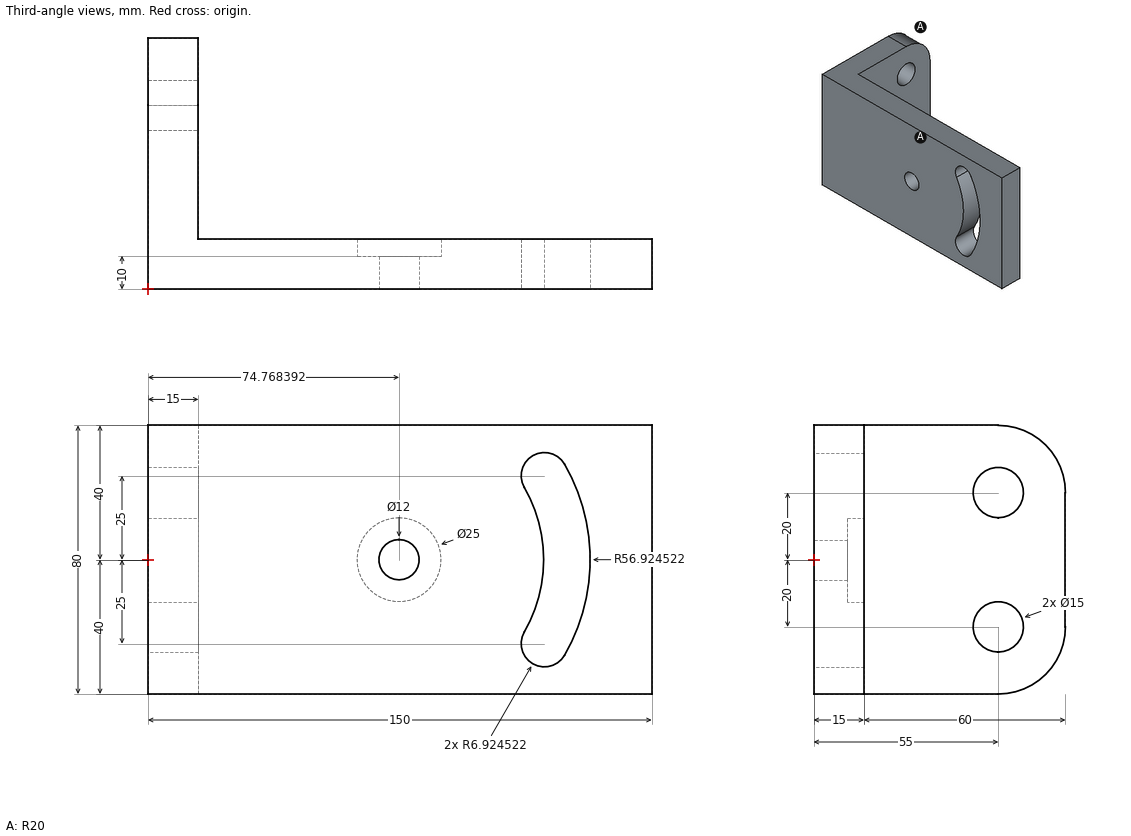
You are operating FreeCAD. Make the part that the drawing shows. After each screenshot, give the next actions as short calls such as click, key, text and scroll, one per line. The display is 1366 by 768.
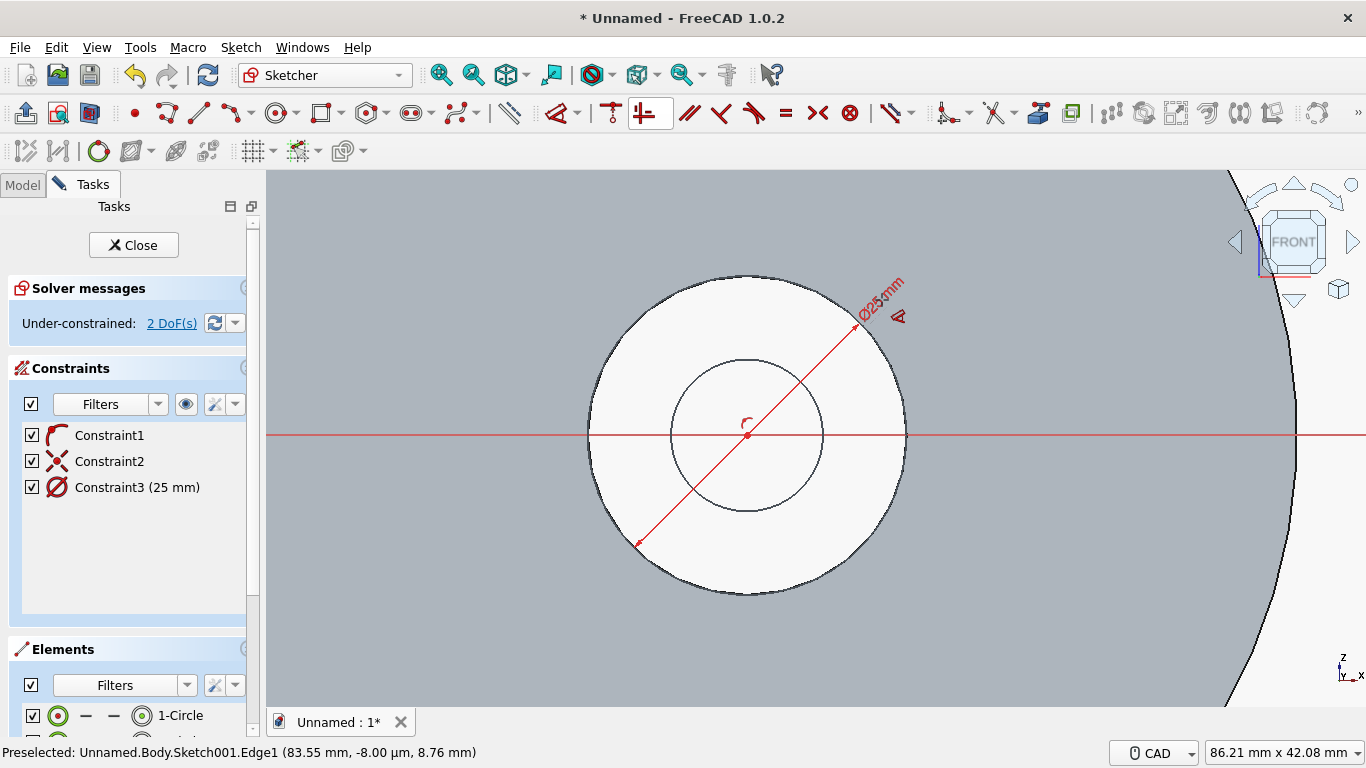
click(801, 382)
click(824, 359)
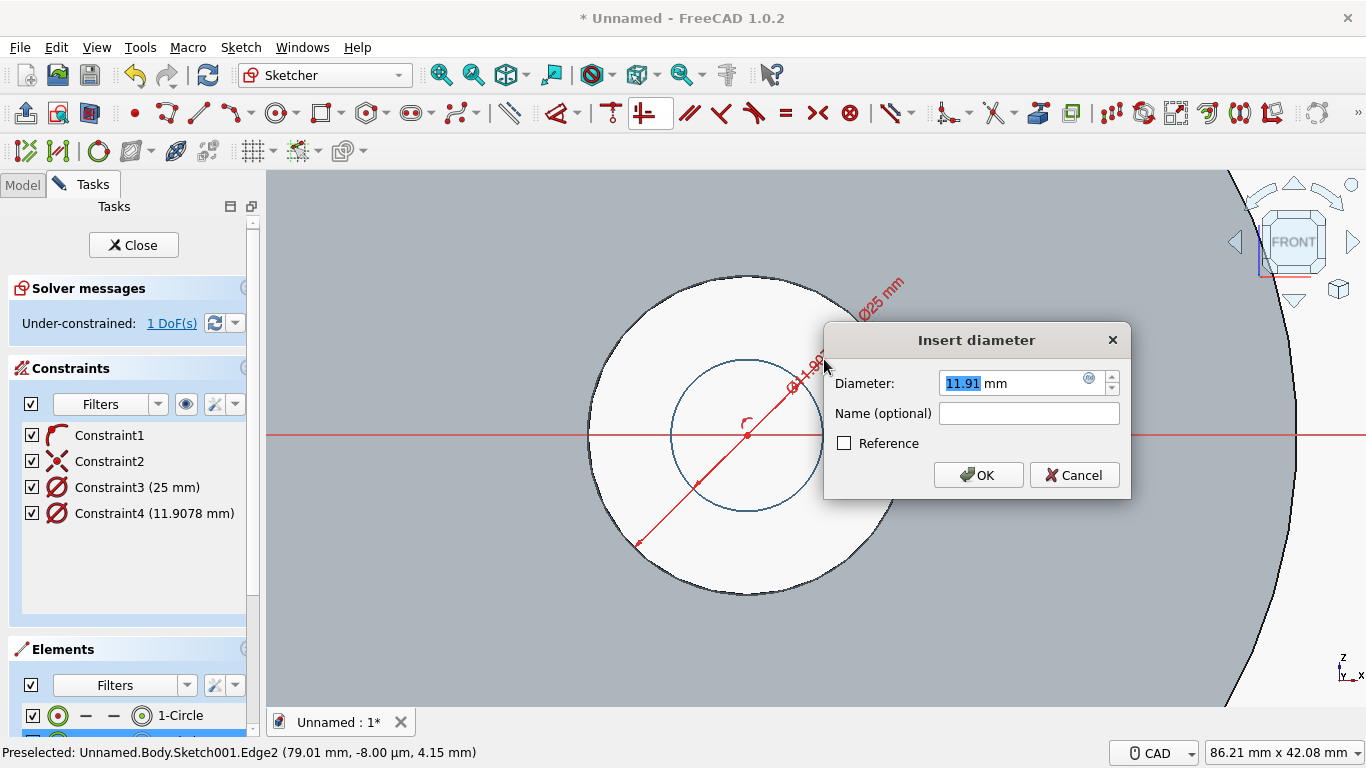
text(12)
key(Return)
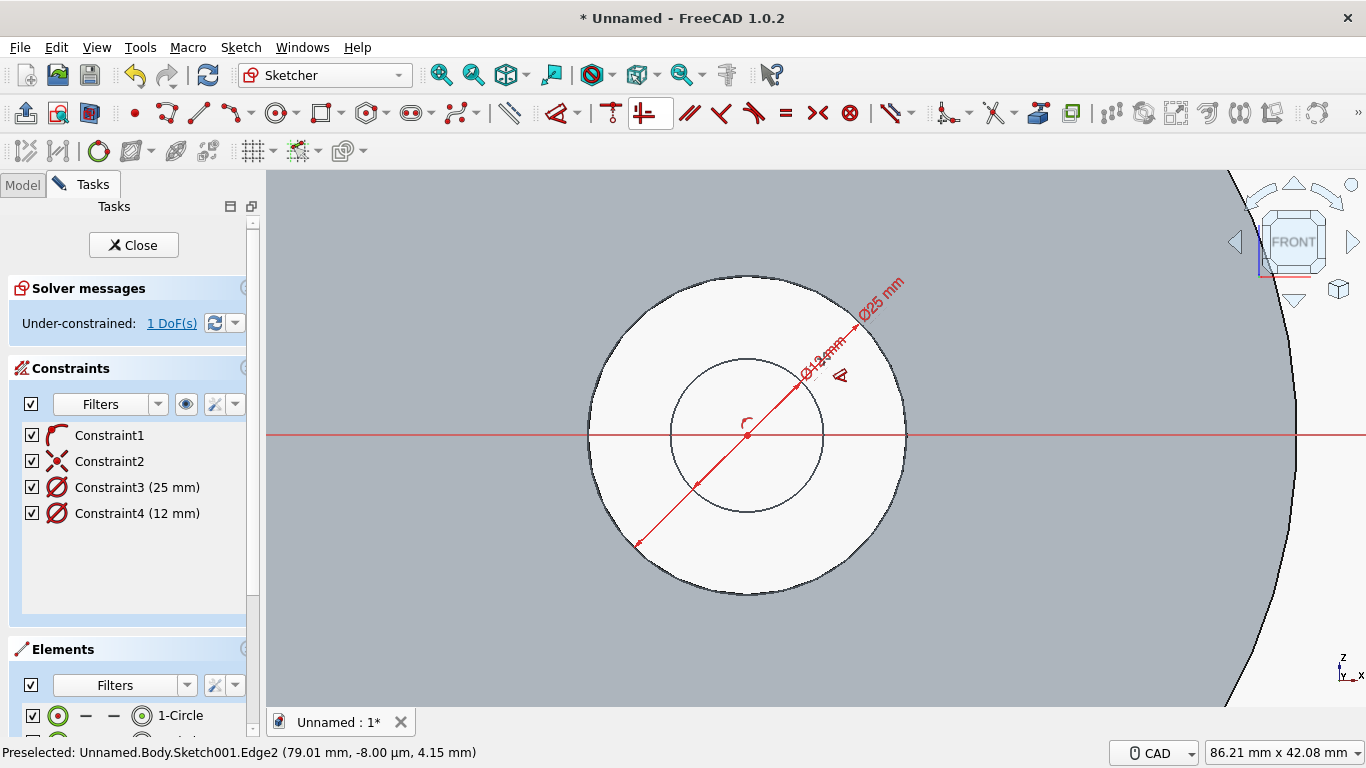
click(747, 435)
click(521, 469)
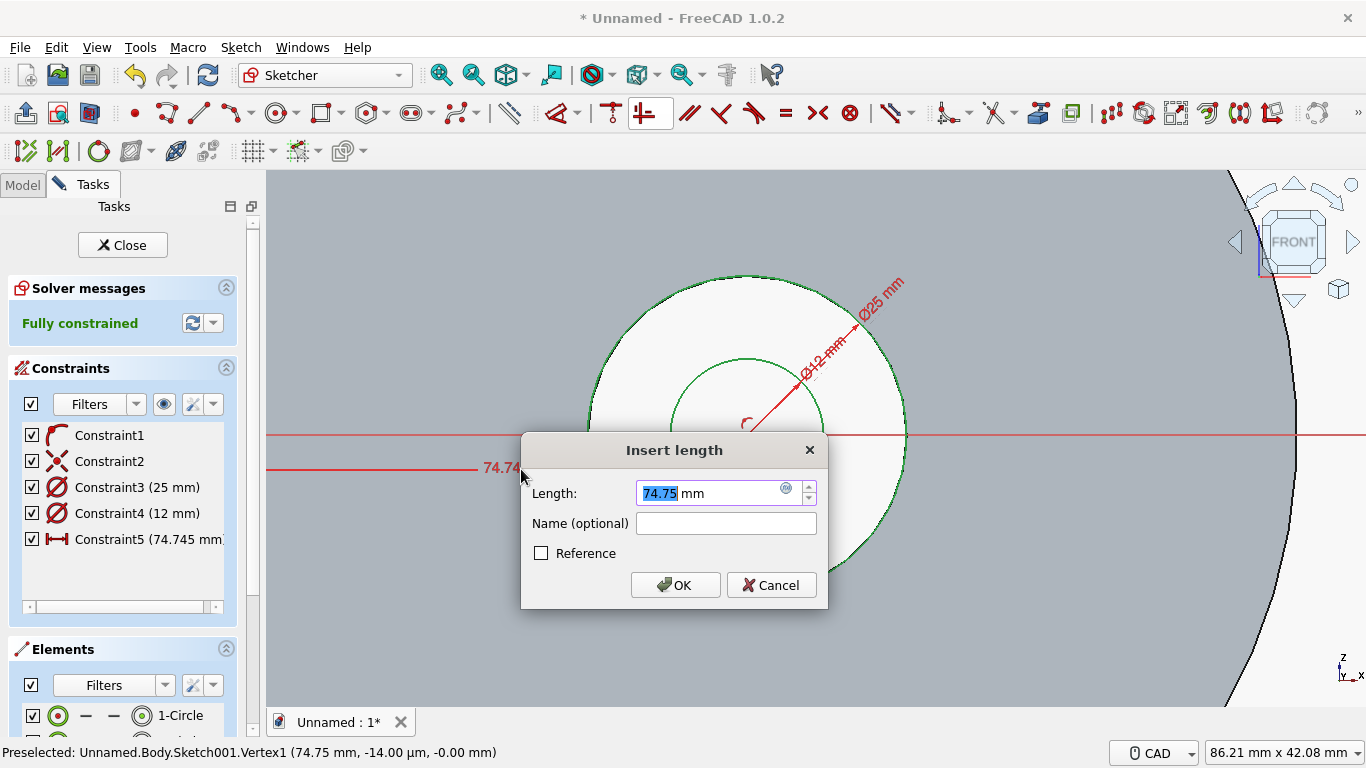
text(74.768392)
key(Return)
key(Escape)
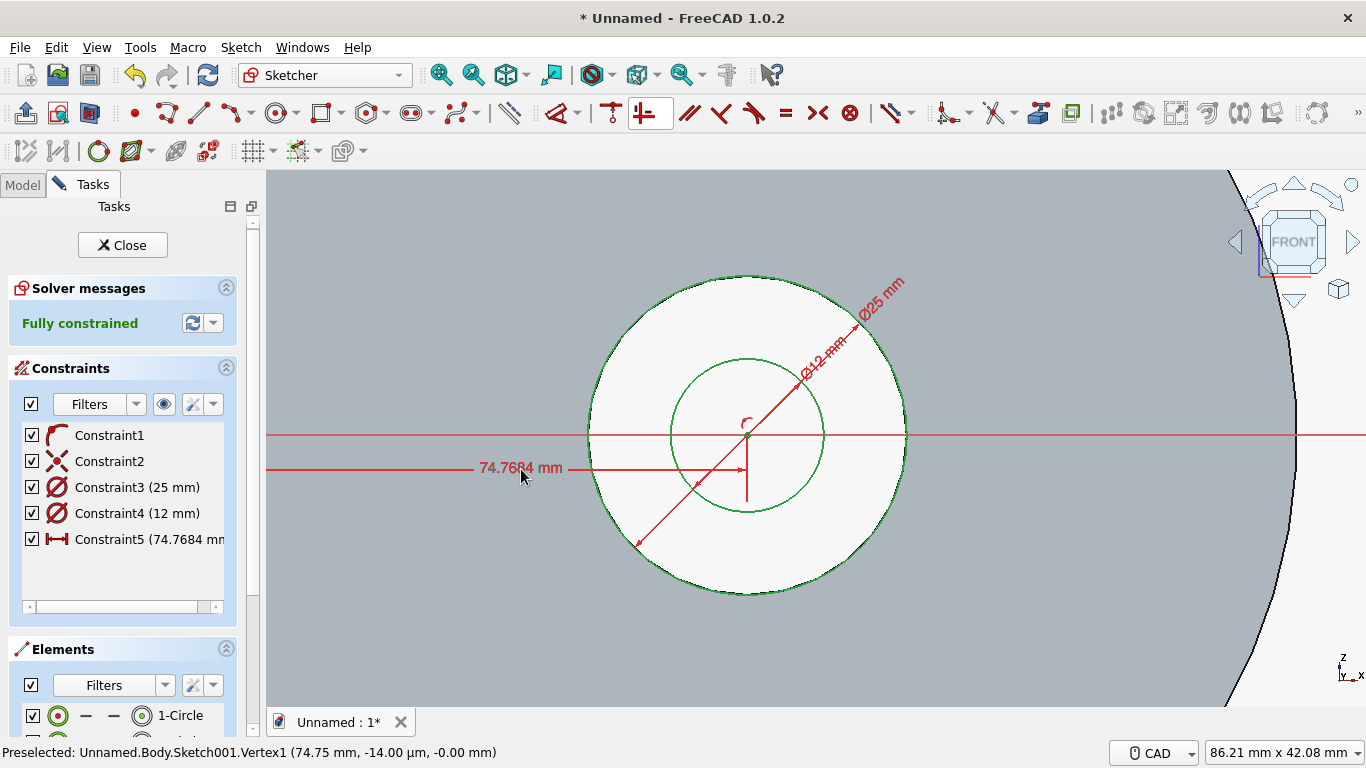
click(123, 245)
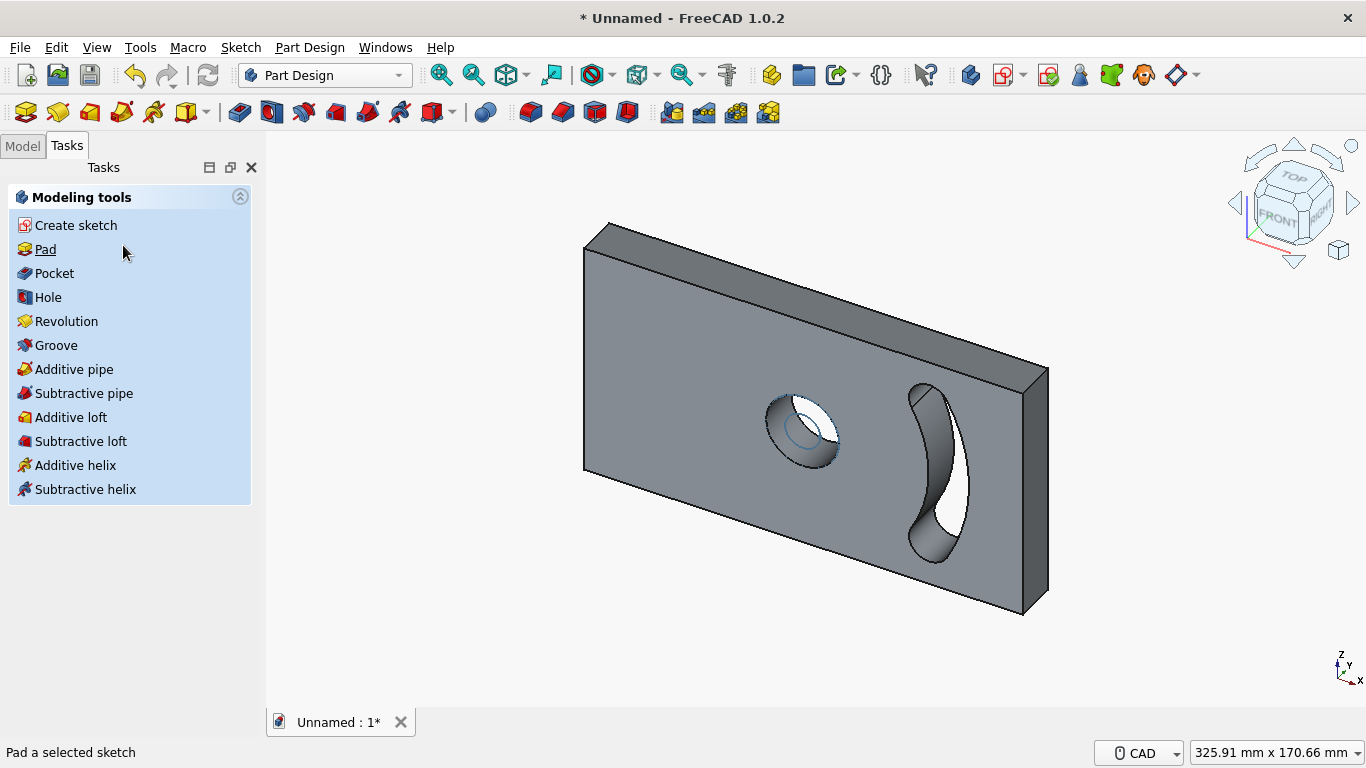
click(26, 112)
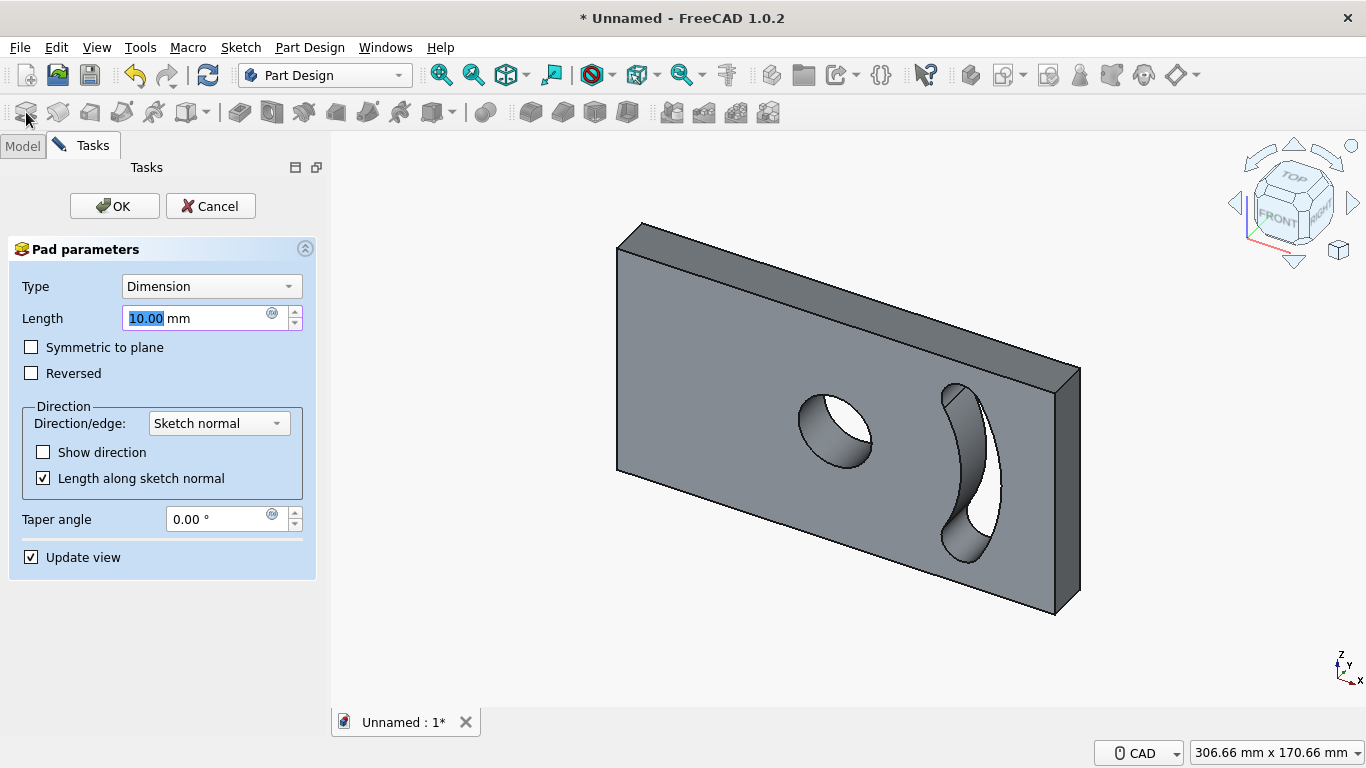
text(10)
key(Tab)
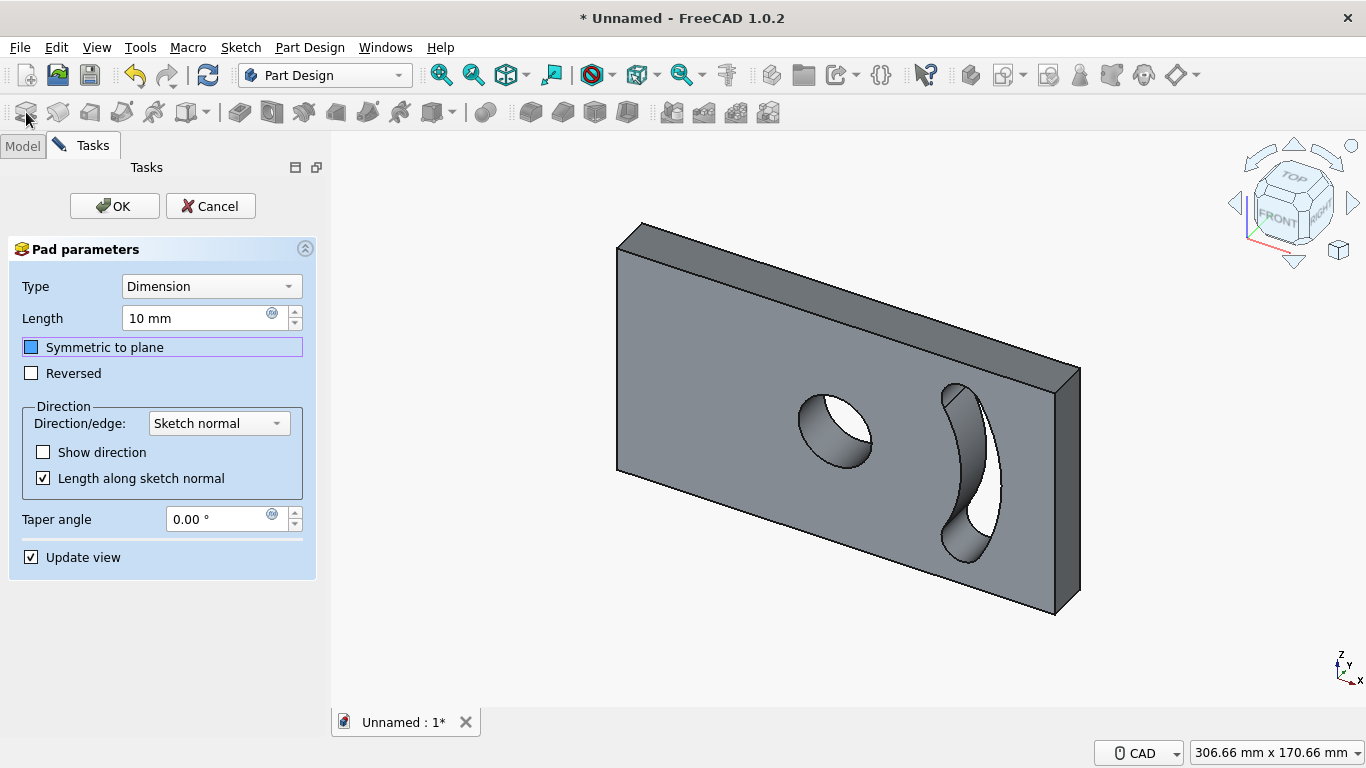
click(30, 373)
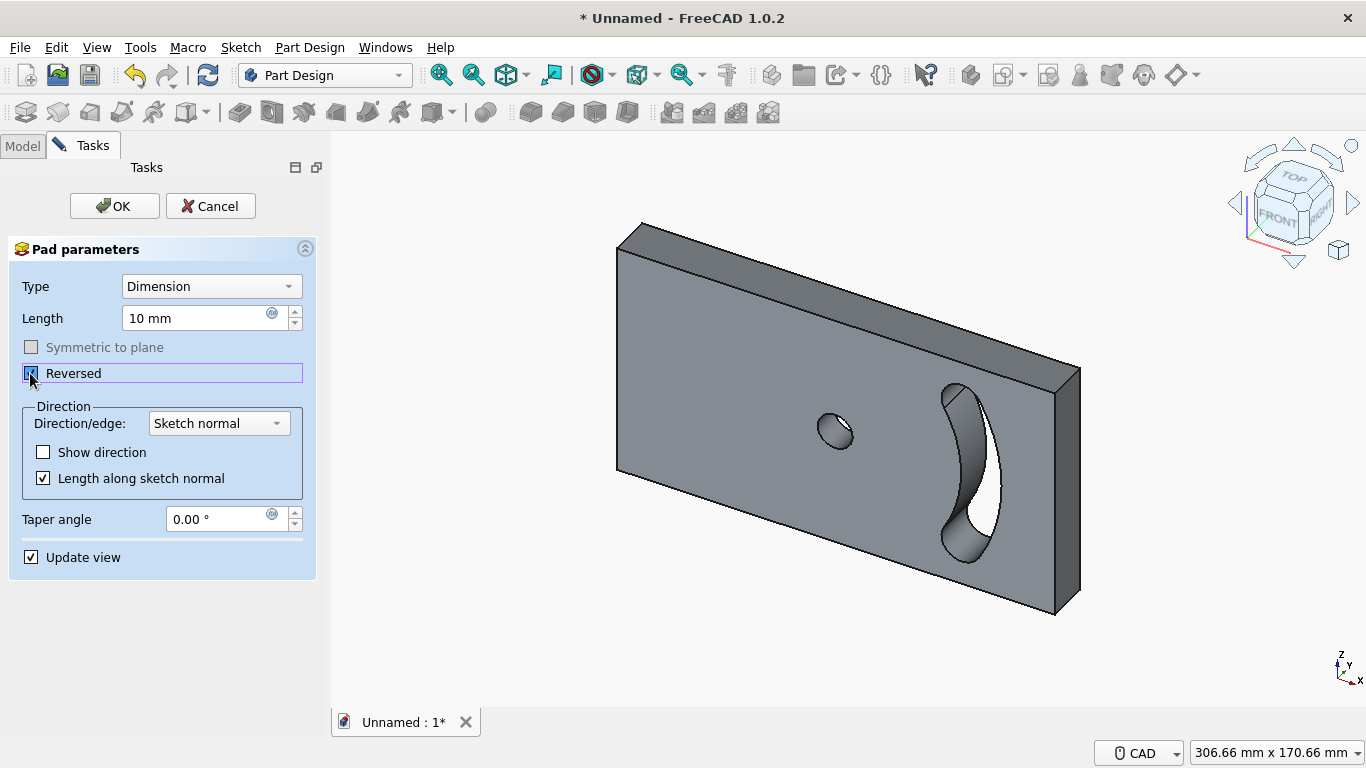
click(115, 206)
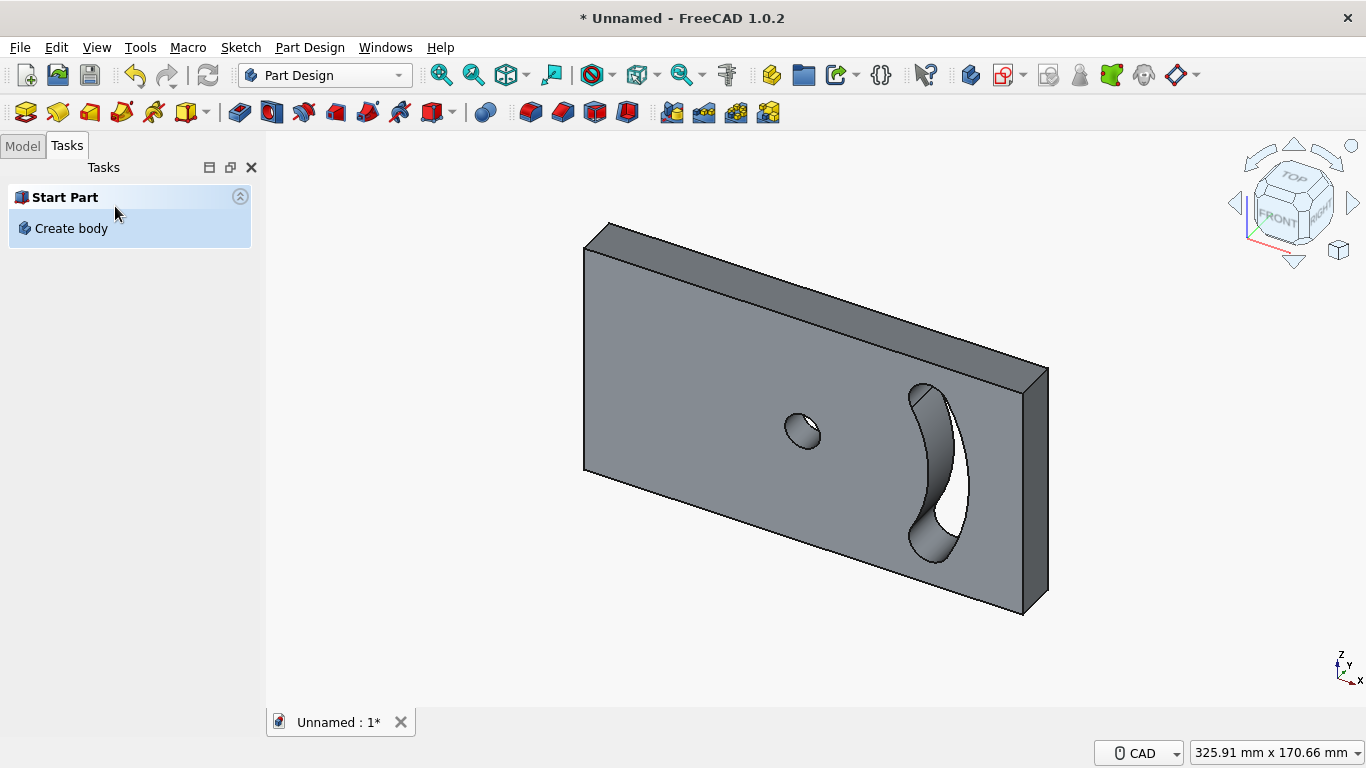
key(4)